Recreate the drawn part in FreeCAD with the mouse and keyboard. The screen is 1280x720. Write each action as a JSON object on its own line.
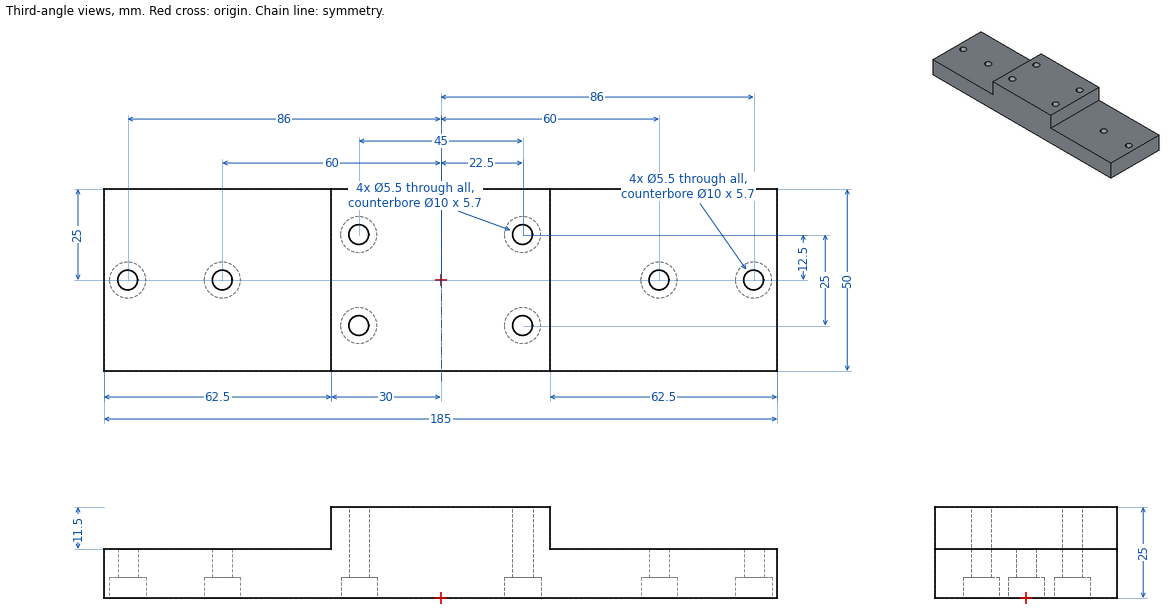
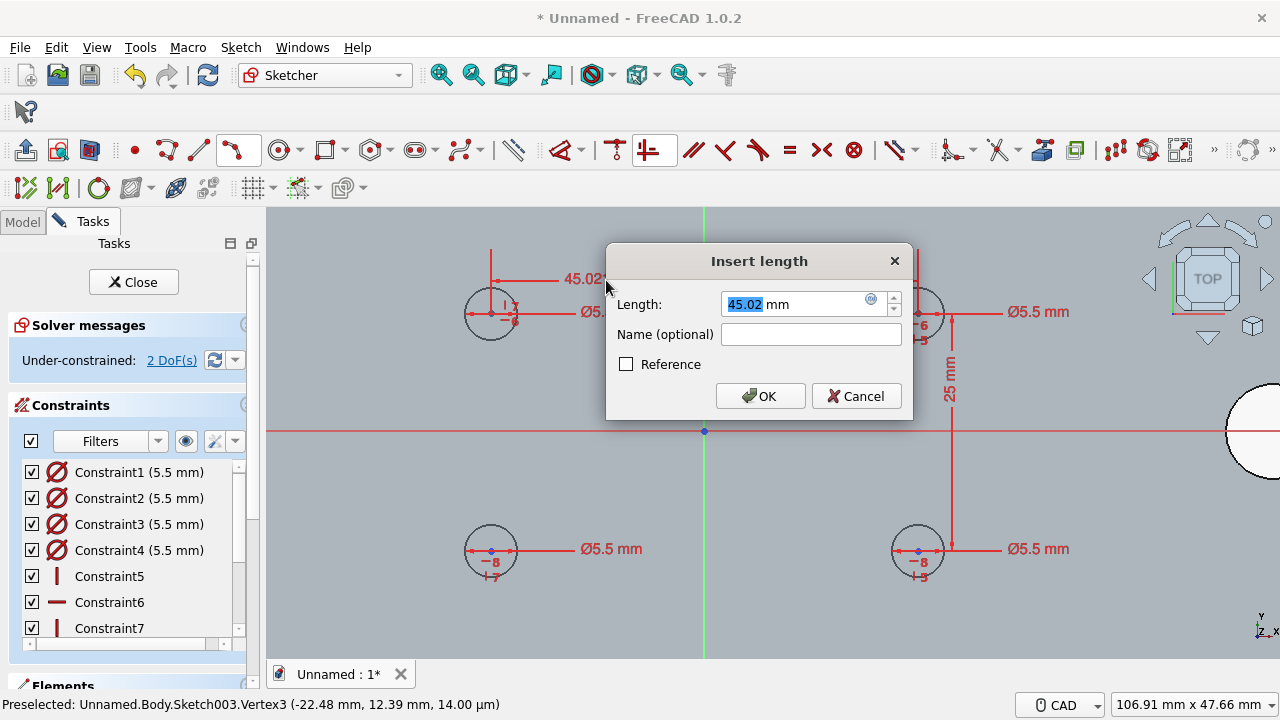
{"action": "type", "text": "45"}
{"action": "key", "text": "Return"}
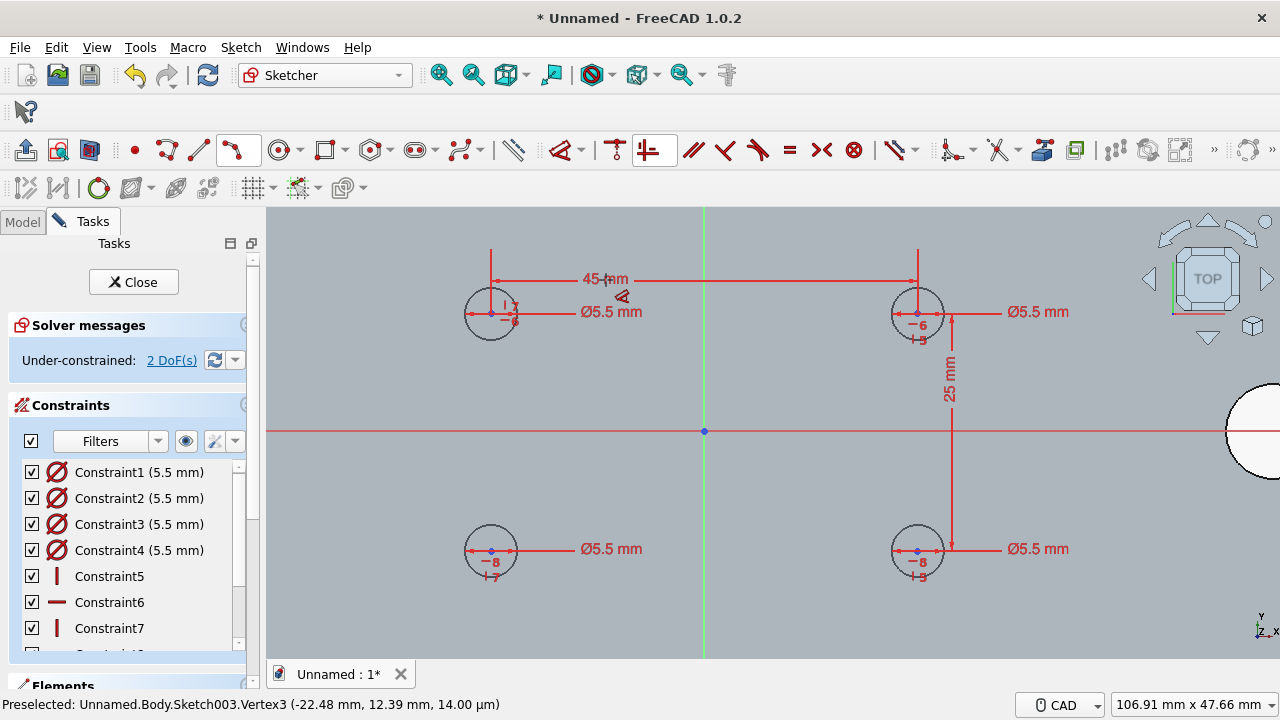
{"action": "left_click", "coordinate": [918, 314]}
{"action": "left_click", "coordinate": [811, 280]}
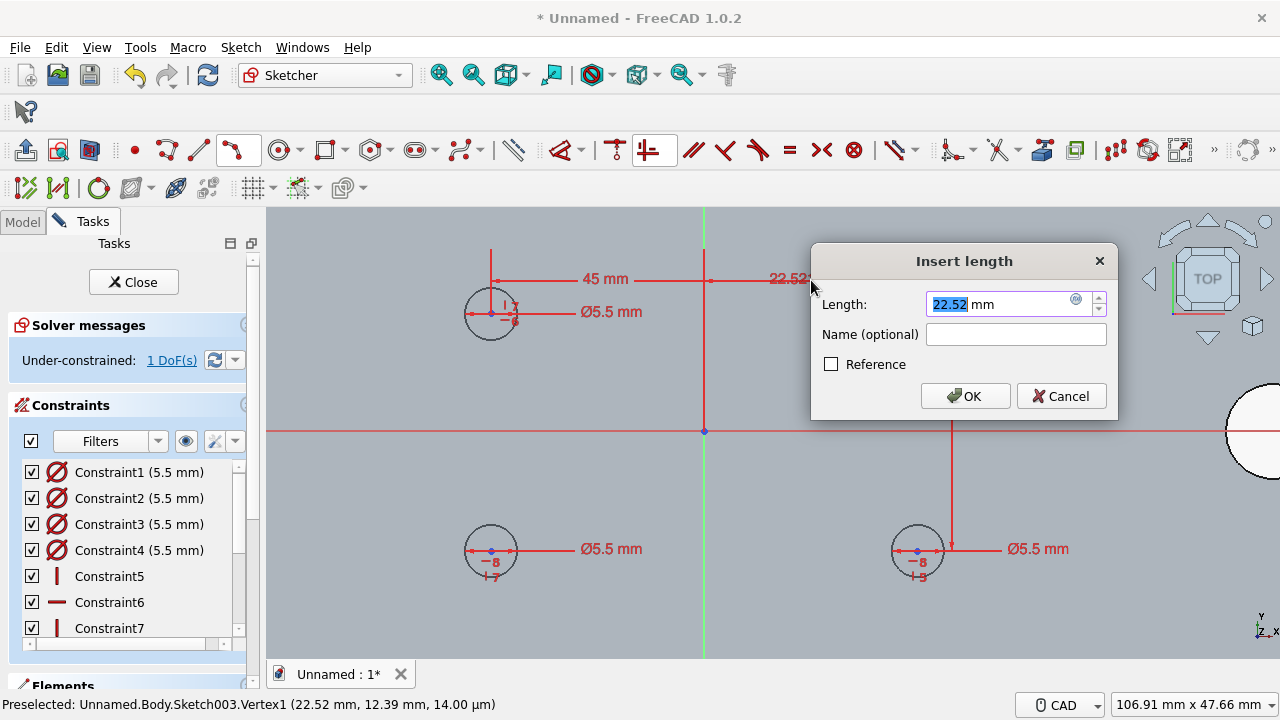
{"action": "type", "text": "22.5"}
{"action": "key", "text": "Return"}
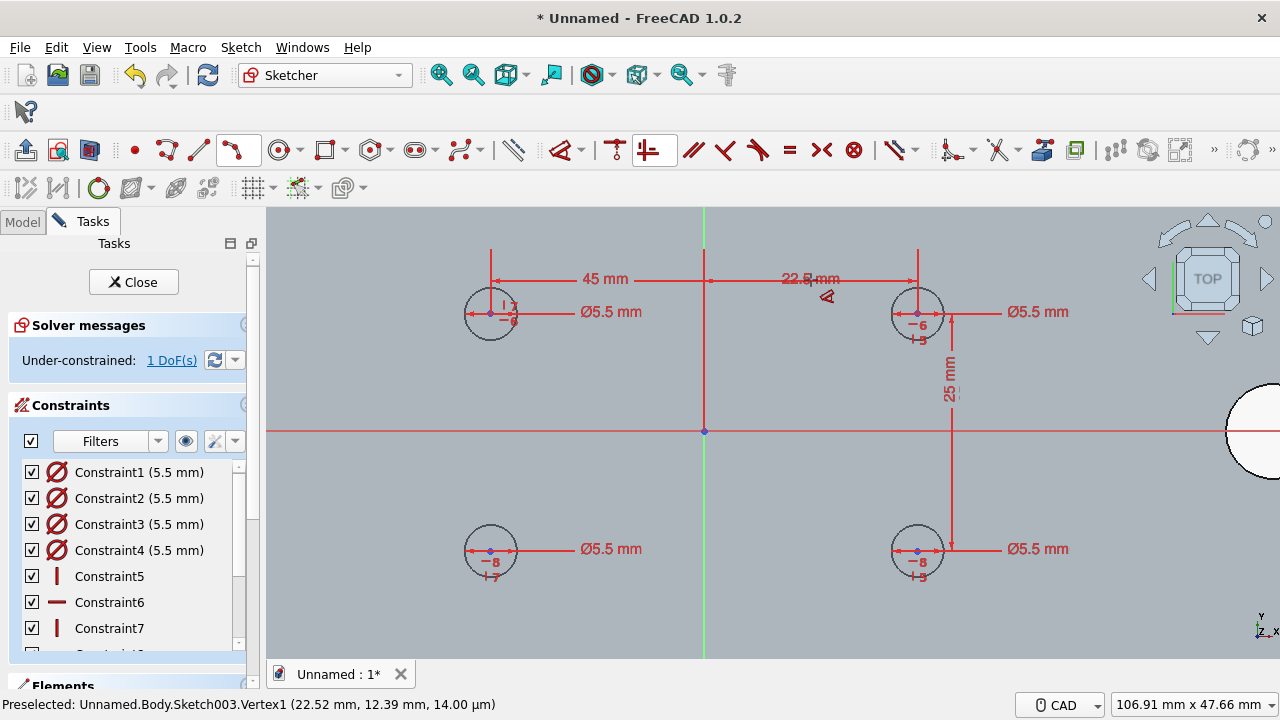
{"action": "left_click", "coordinate": [918, 314]}
{"action": "left_click", "coordinate": [952, 346]}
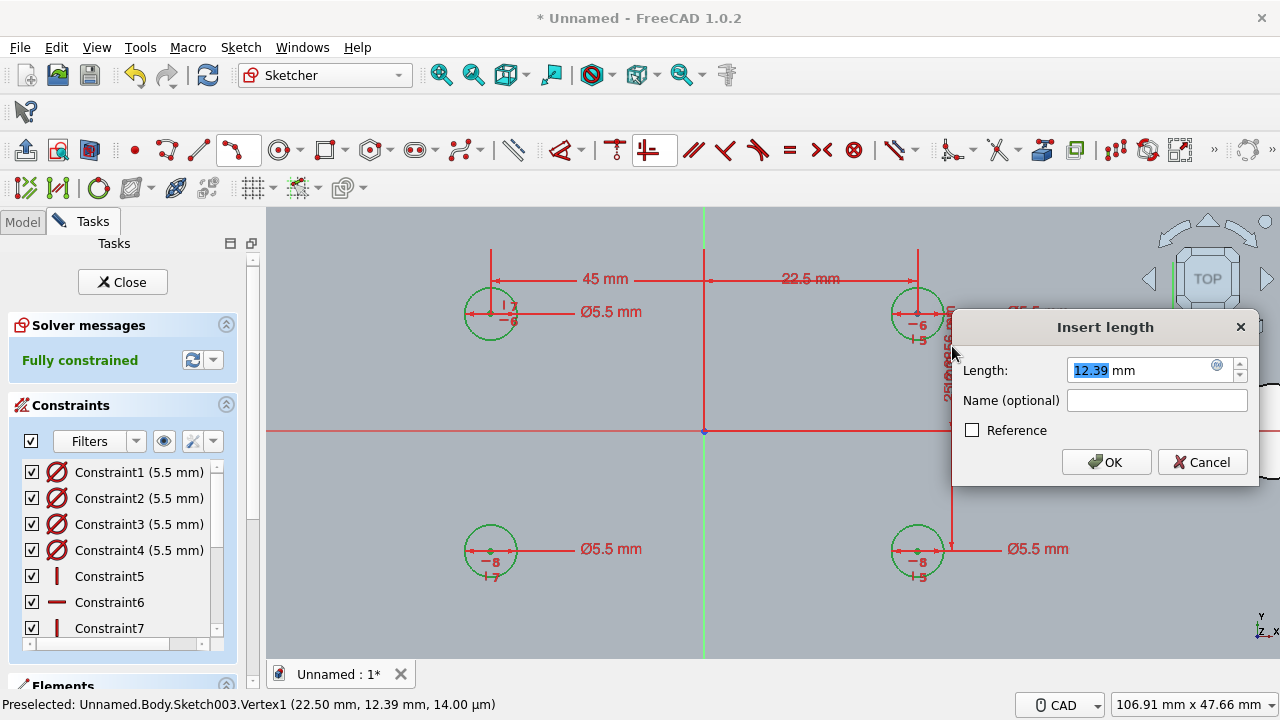
{"action": "type", "text": "12.5"}
{"action": "key", "text": "Return"}
{"action": "key", "text": "Escape"}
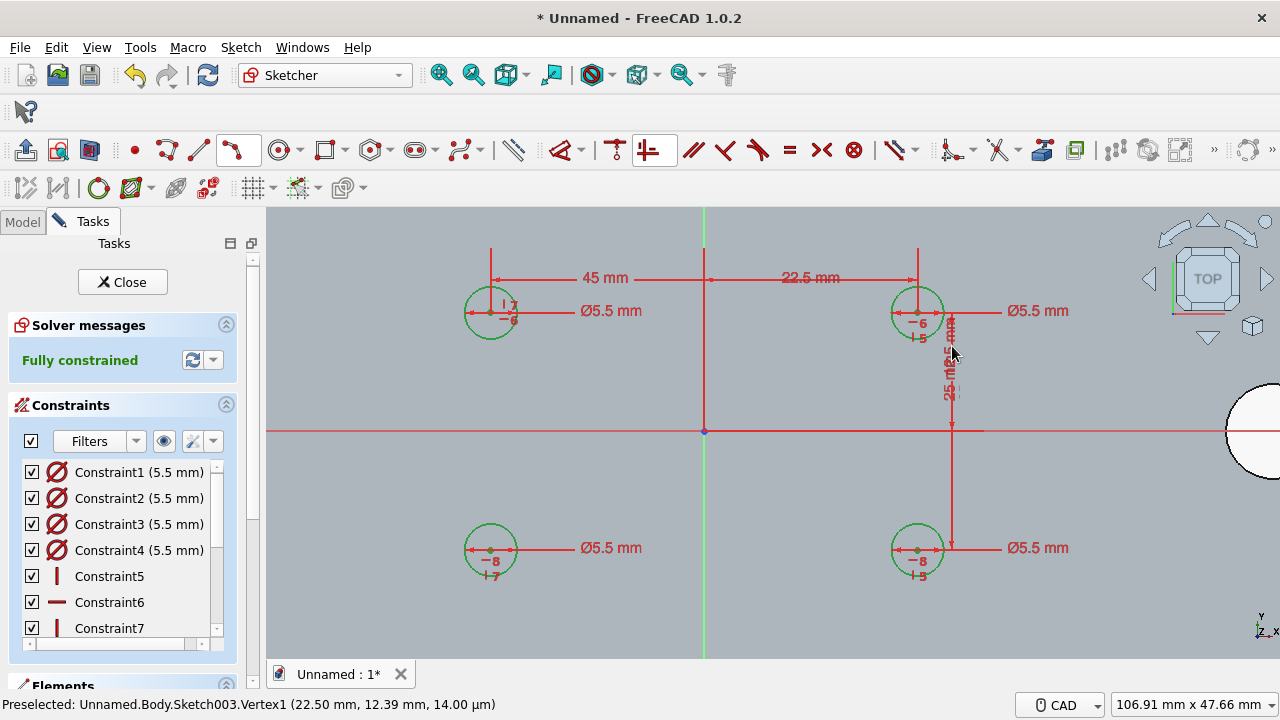
{"action": "left_click", "coordinate": [123, 282]}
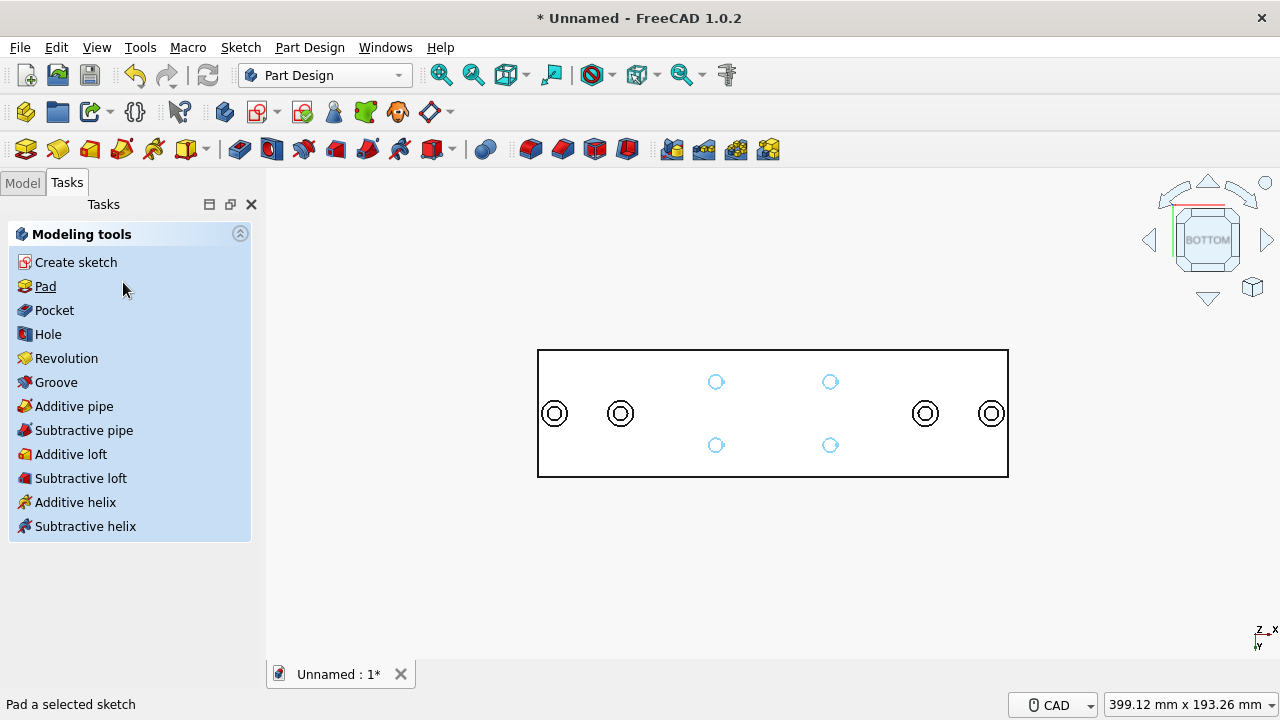
{"action": "left_click", "coordinate": [272, 150]}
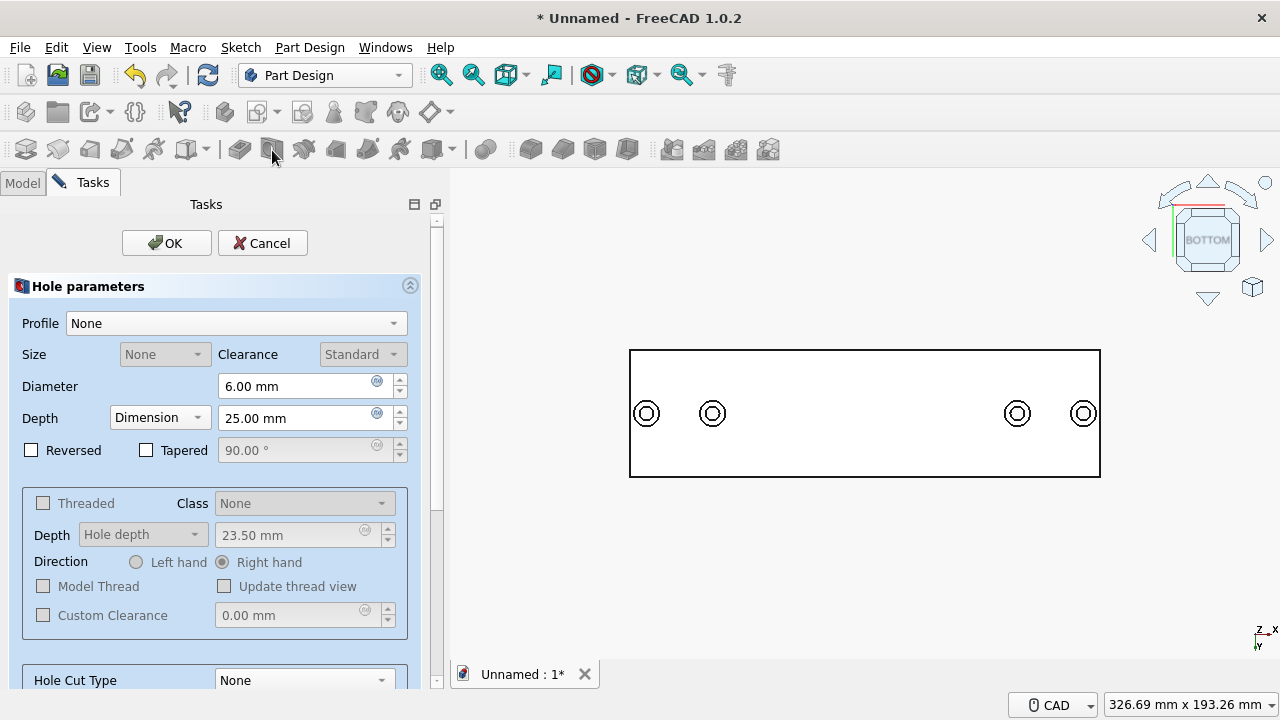
{"action": "triple_click", "coordinate": [305, 386]}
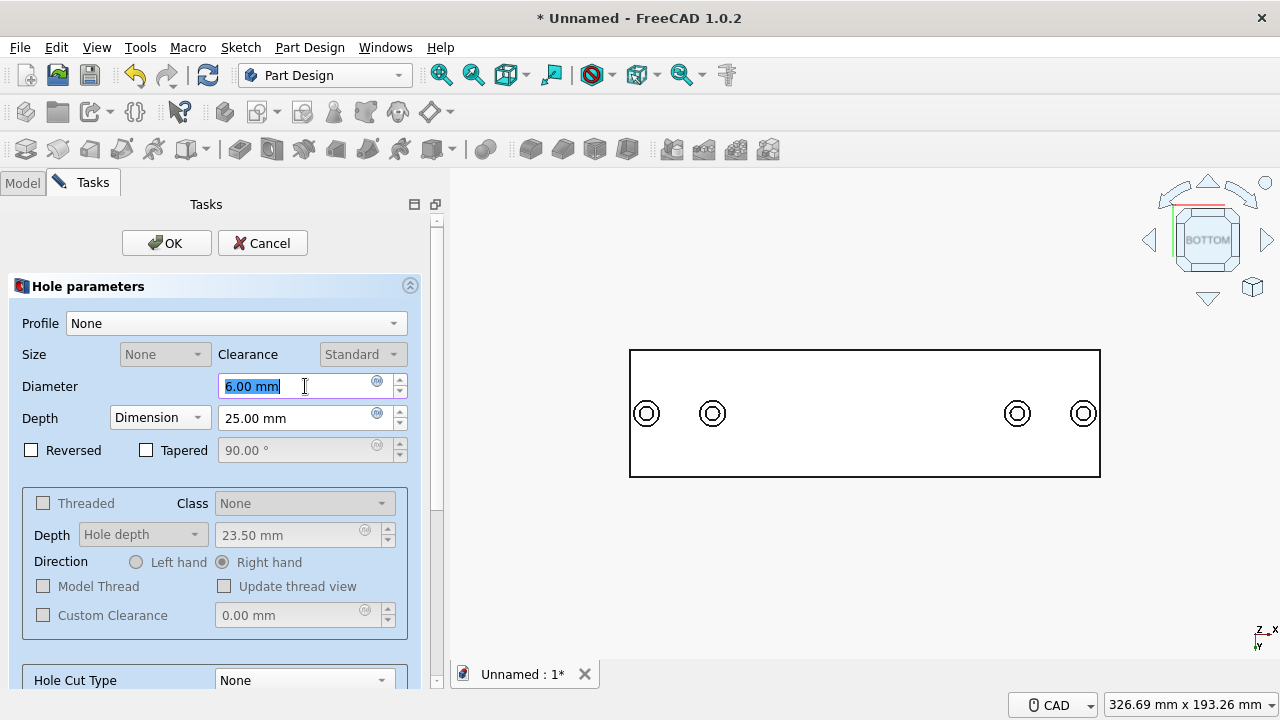
{"action": "type", "text": "5.5"}
{"action": "key", "text": "Tab"}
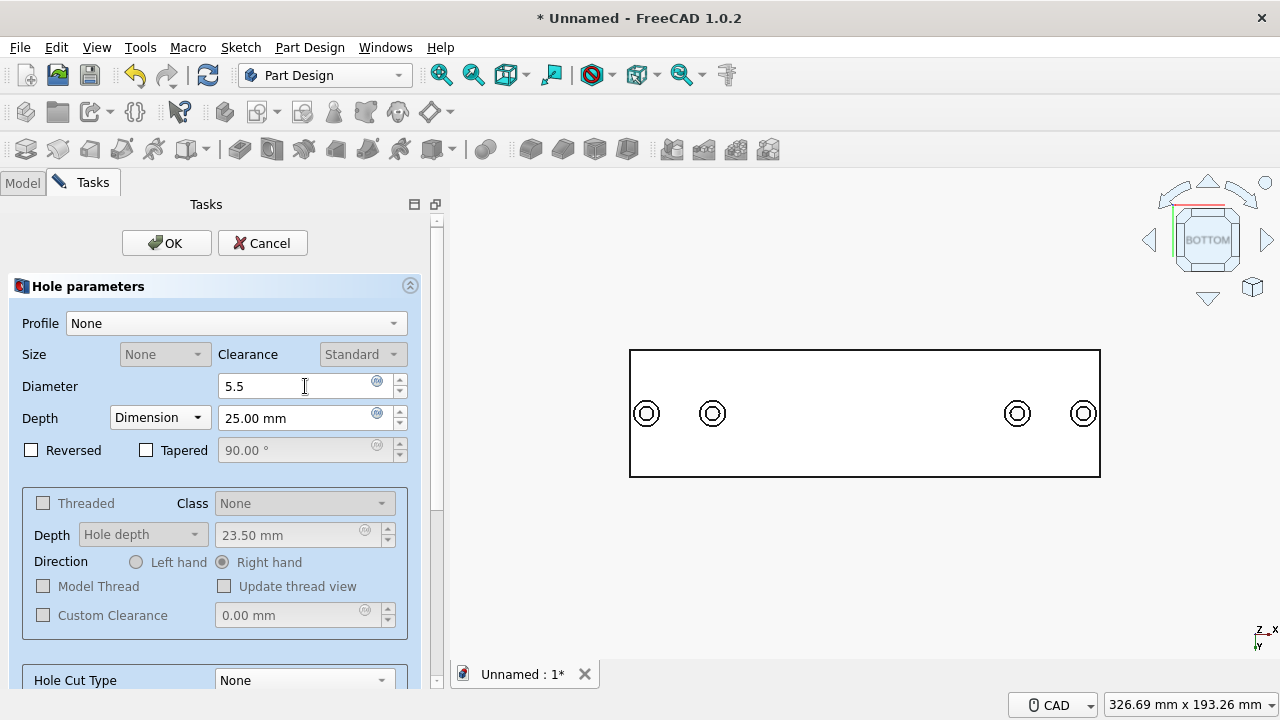
{"action": "left_click", "coordinate": [161, 418]}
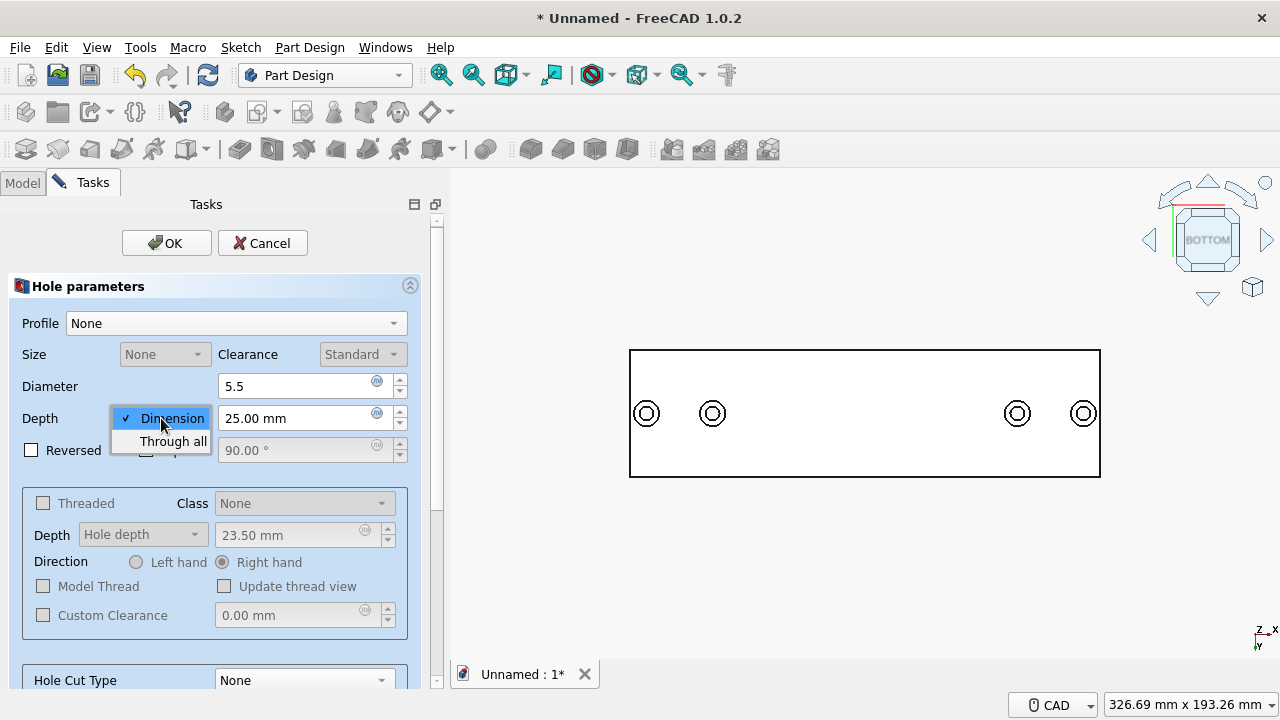
{"action": "left_click", "coordinate": [160, 442]}